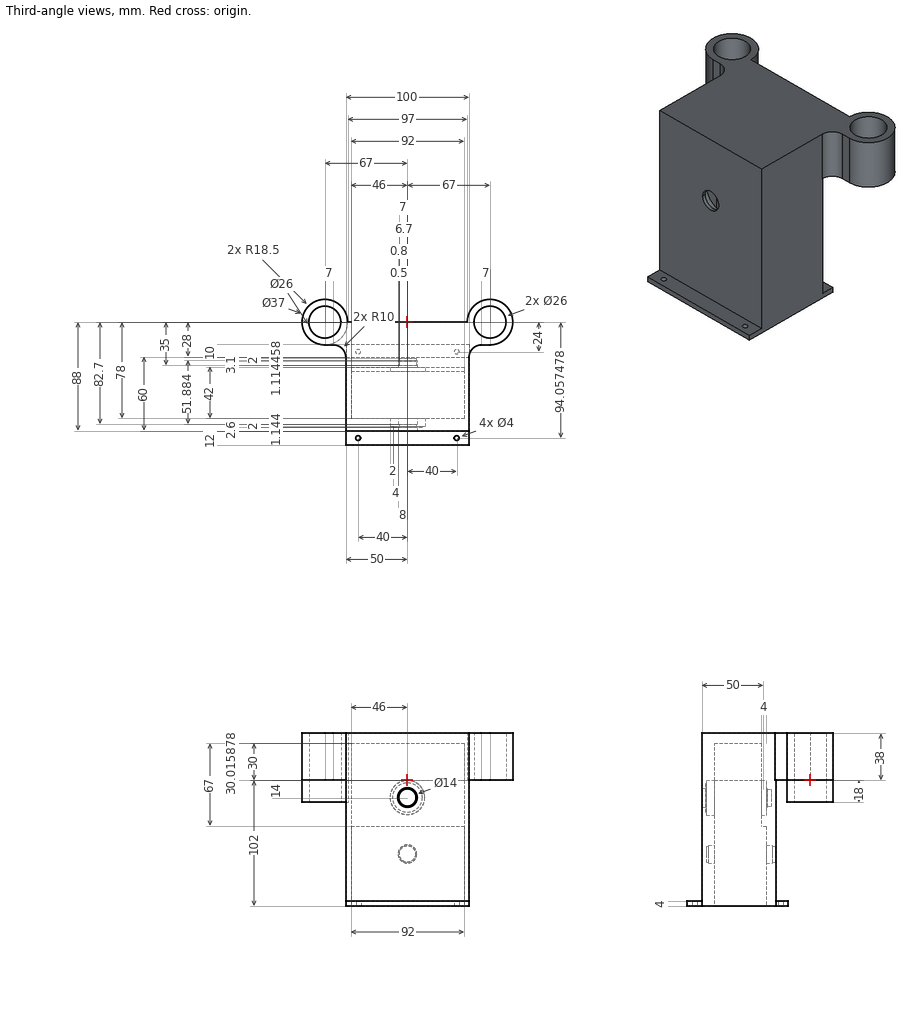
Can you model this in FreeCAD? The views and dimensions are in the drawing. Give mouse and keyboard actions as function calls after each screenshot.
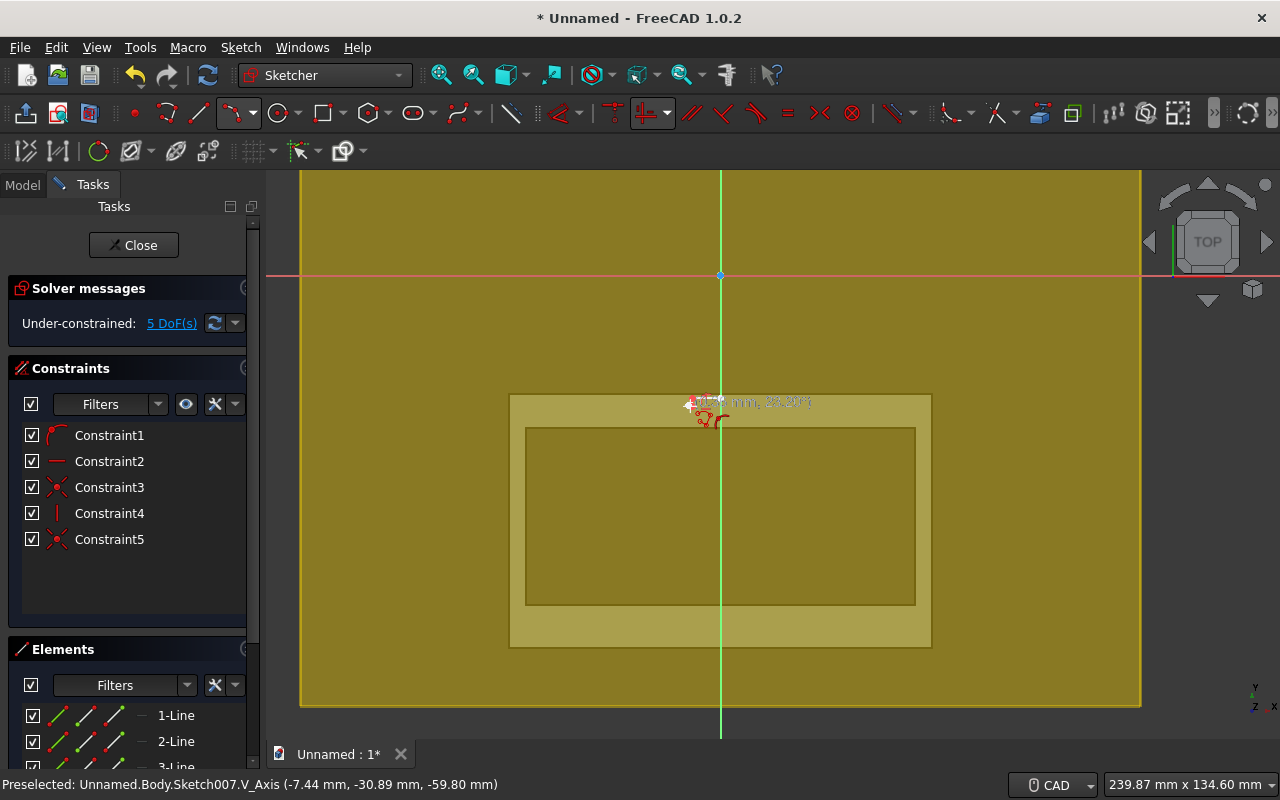
click(689, 625)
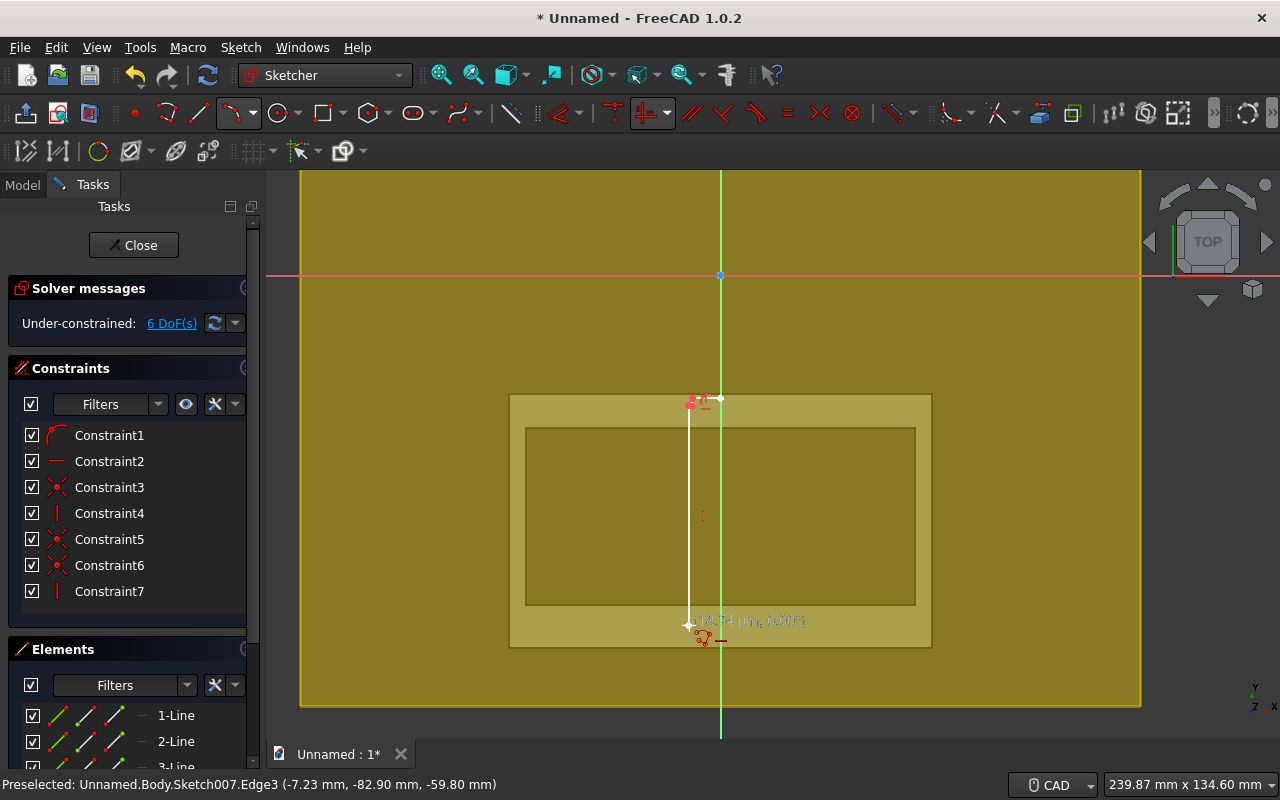
scroll(692, 625, up, 8)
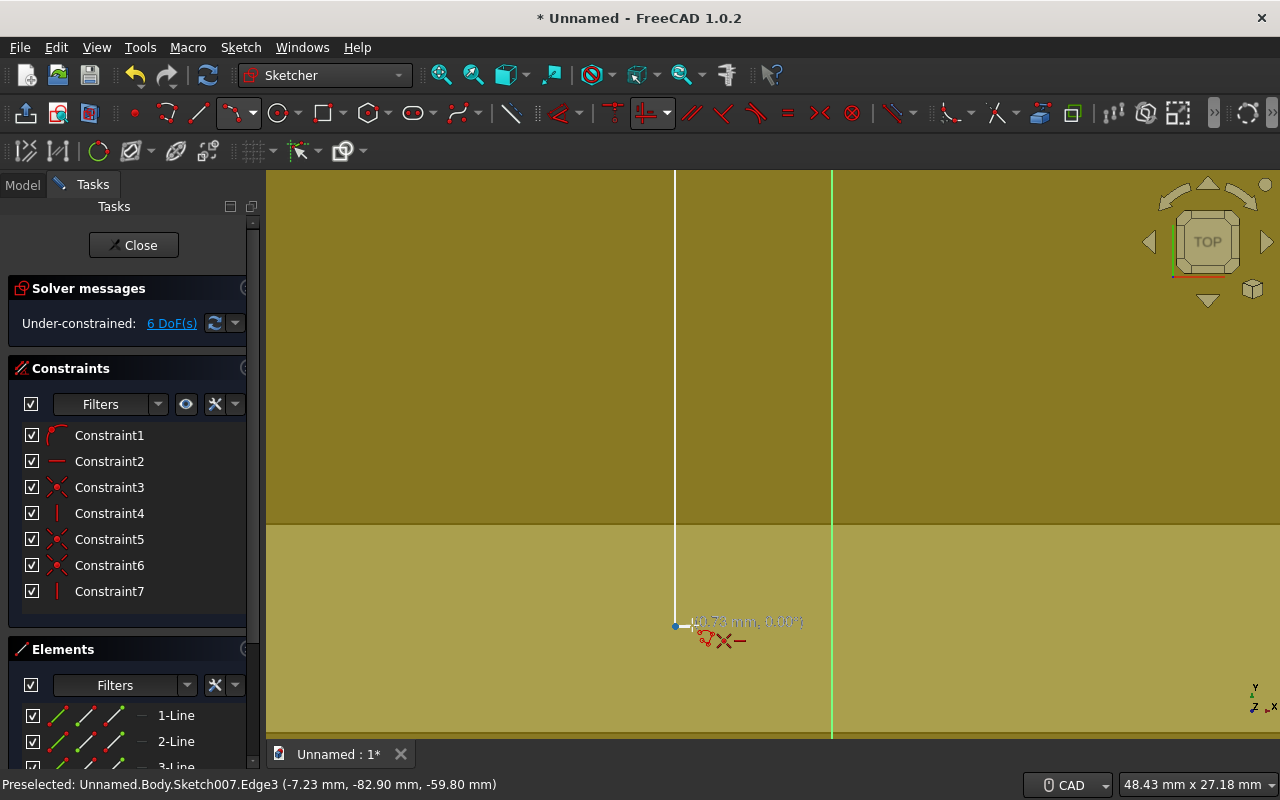
click(692, 622)
click(692, 664)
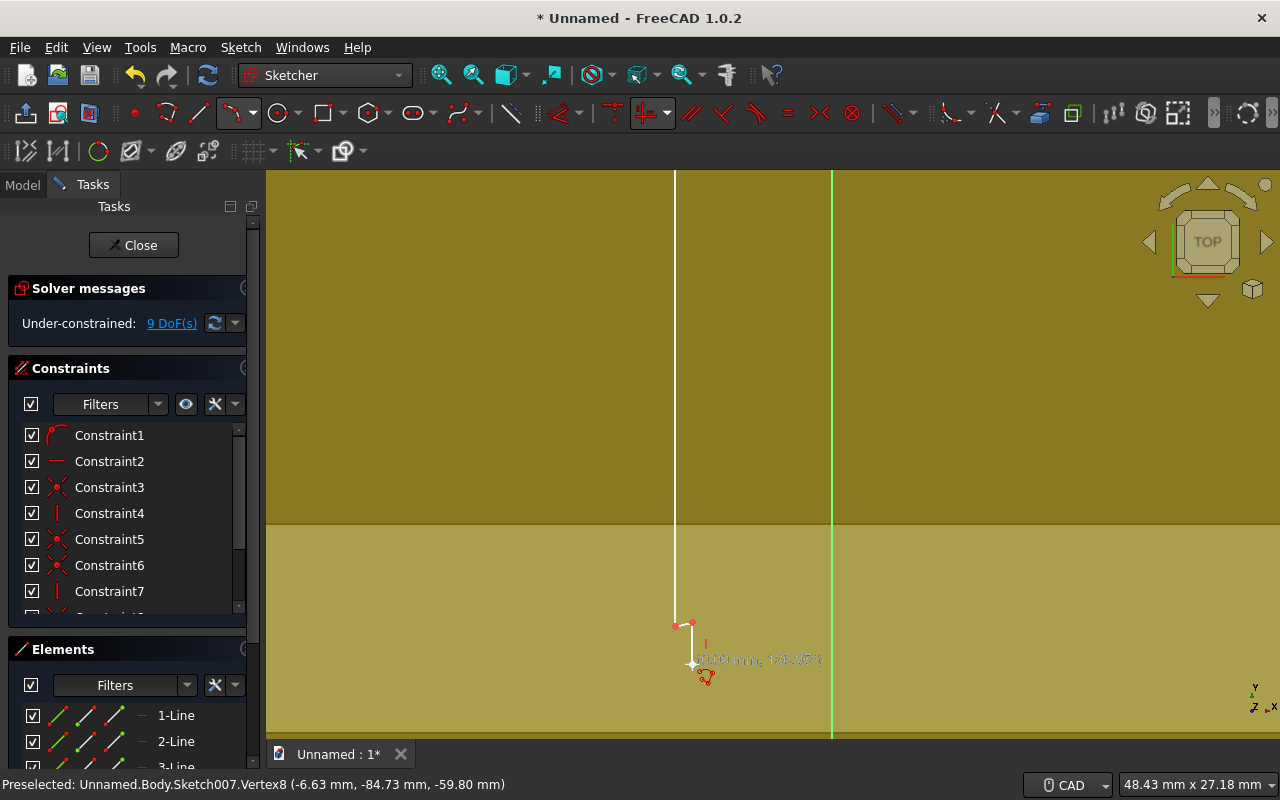
scroll(692, 626, down, 8)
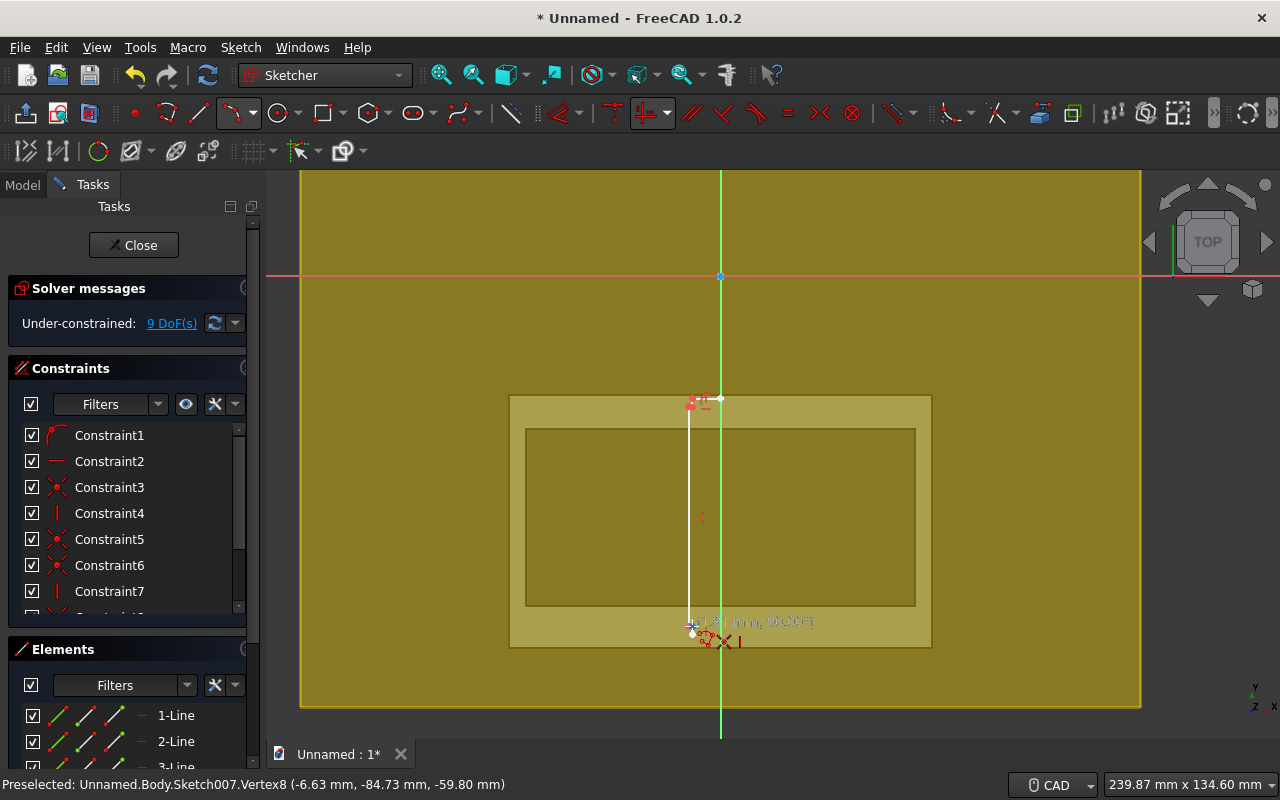
click(712, 634)
click(721, 399)
key(Escape)
key(Escape)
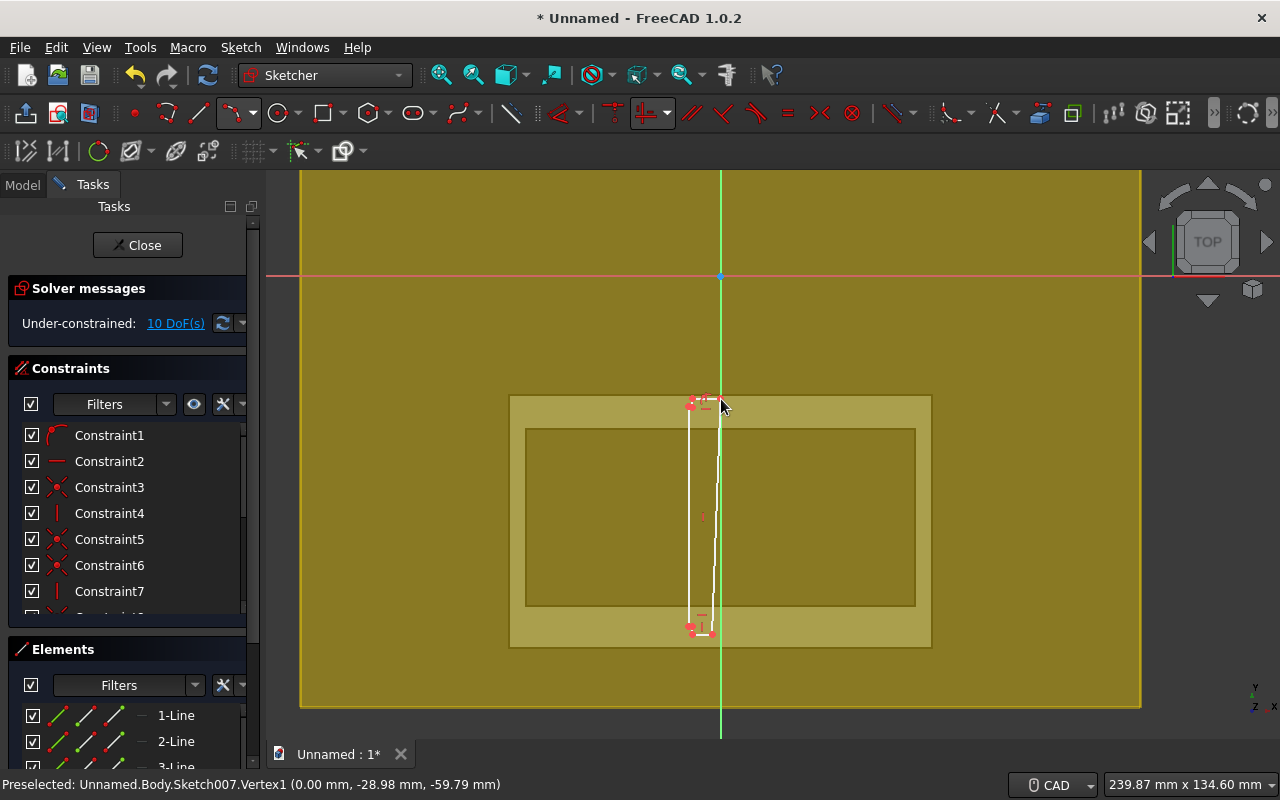
scroll(691, 407, up, 11)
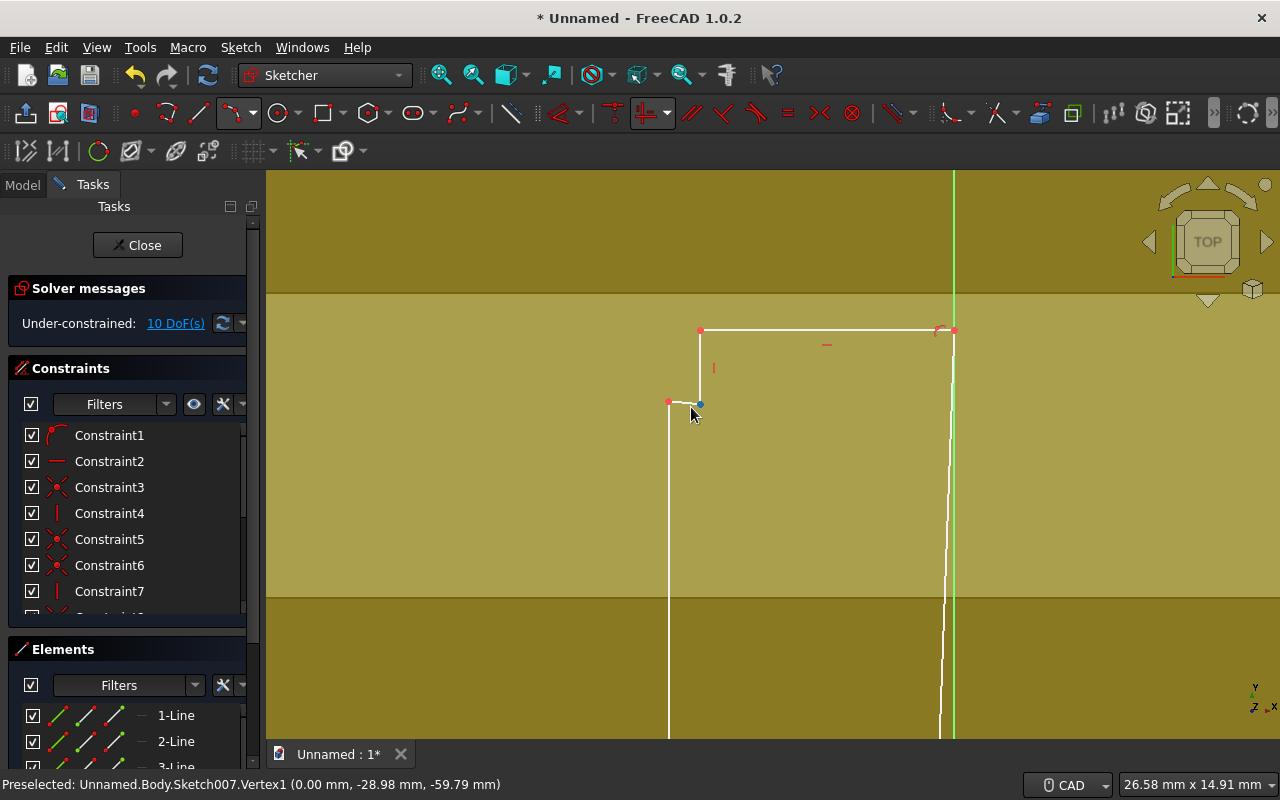
click(684, 403)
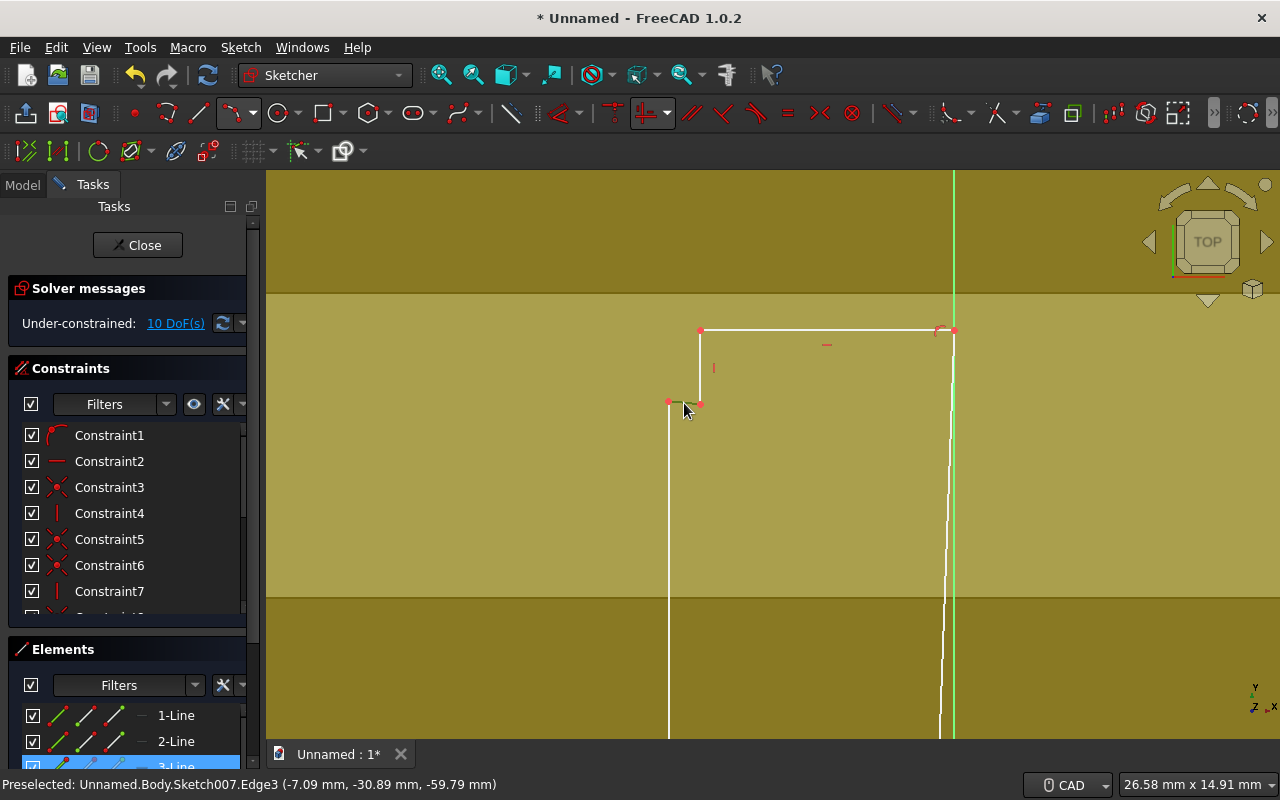
key(h)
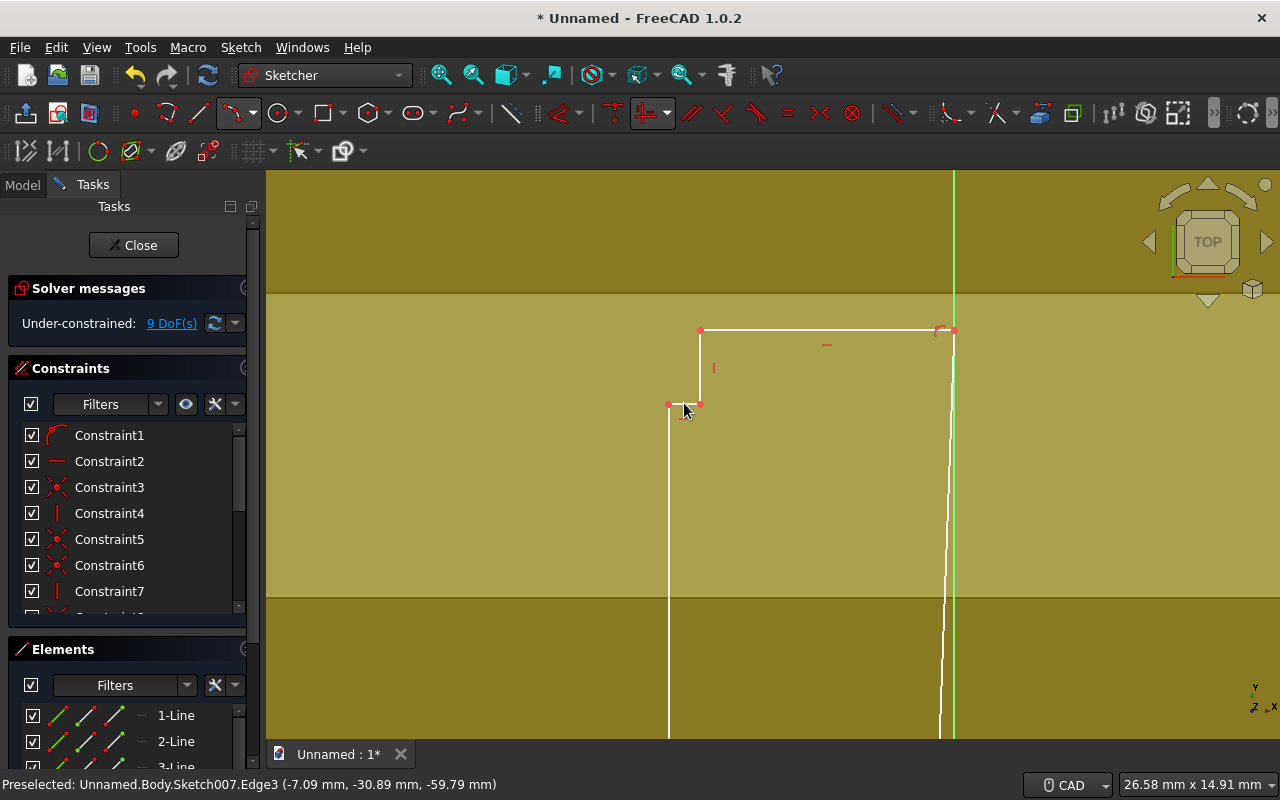
scroll(691, 406, down, 11)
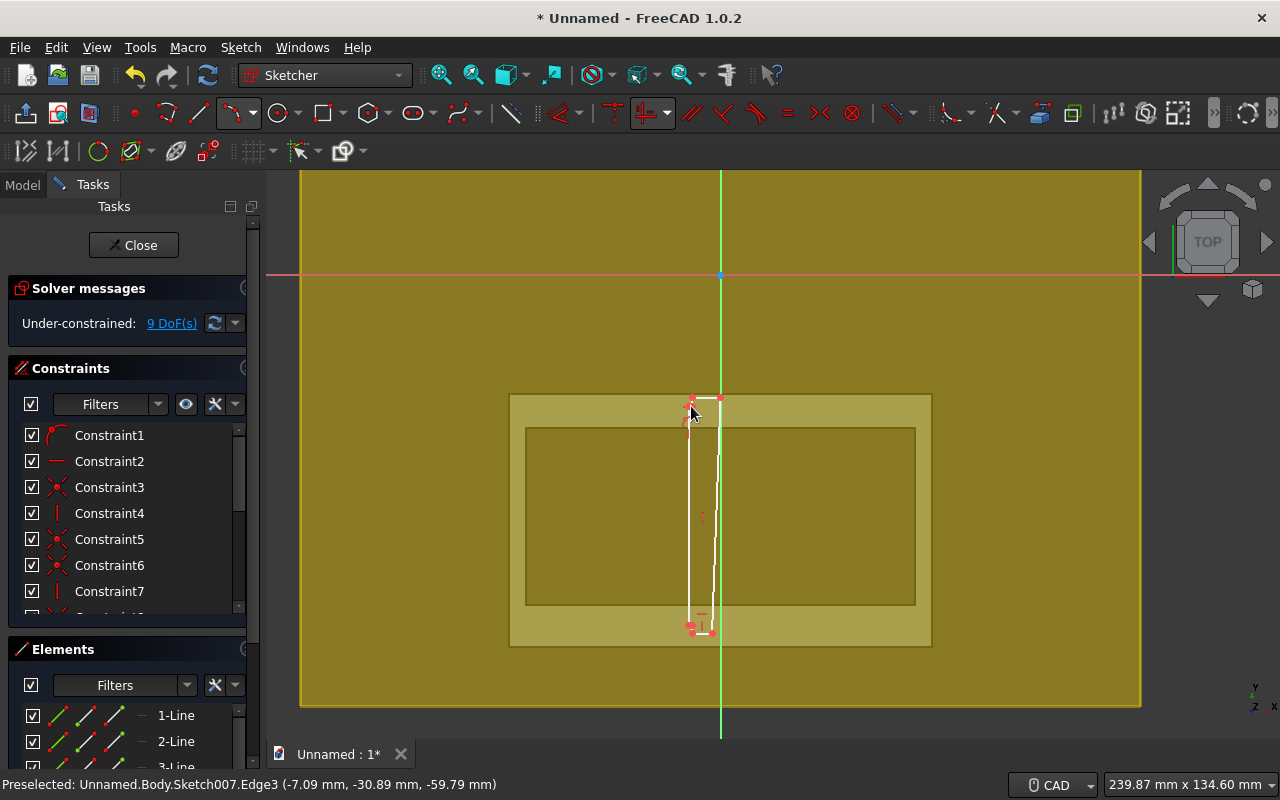
scroll(690, 626, up, 14)